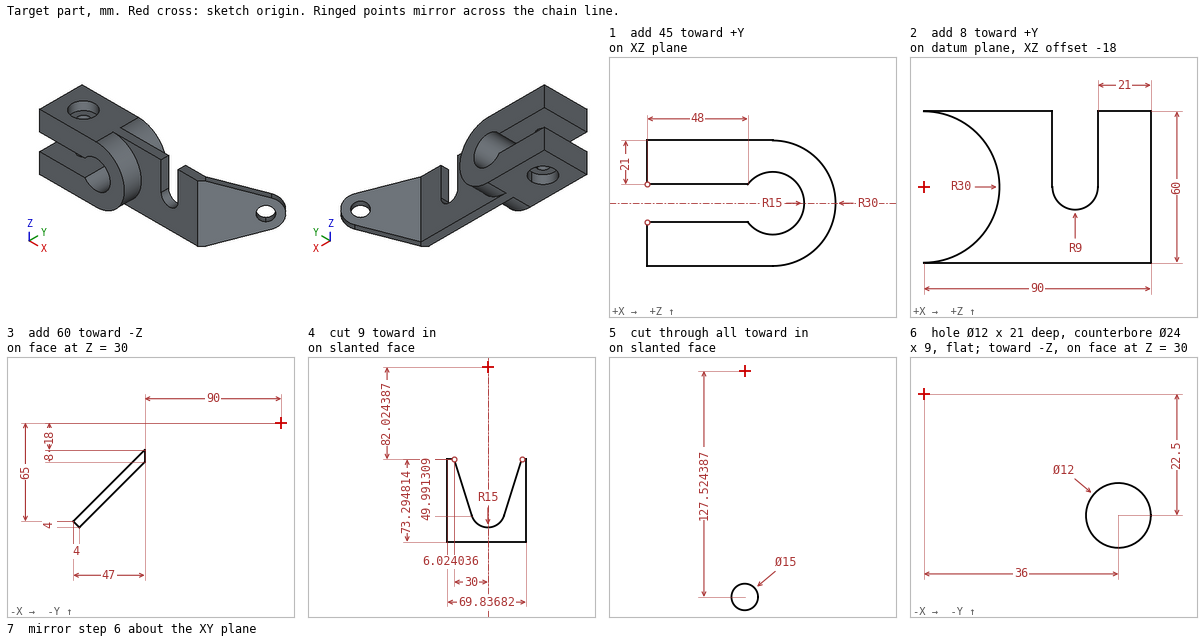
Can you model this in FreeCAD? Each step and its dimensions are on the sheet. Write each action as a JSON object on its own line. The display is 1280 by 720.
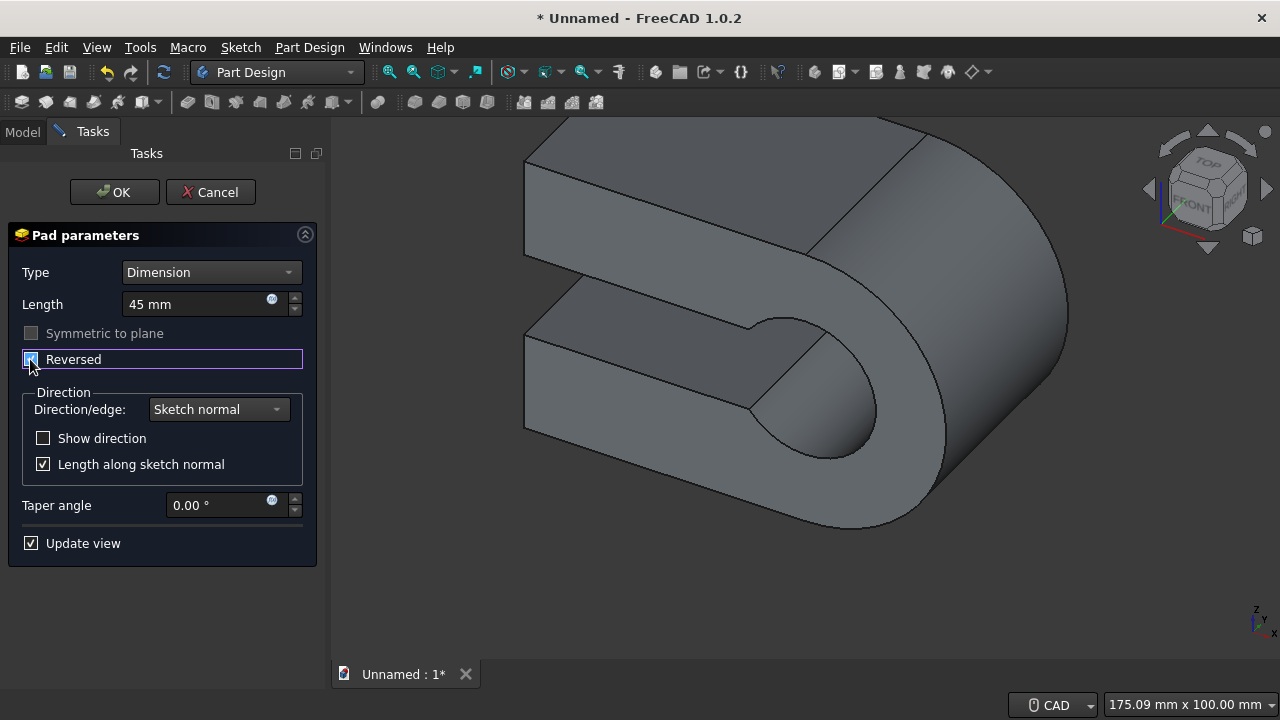
{"action": "left_click", "coordinate": [115, 192]}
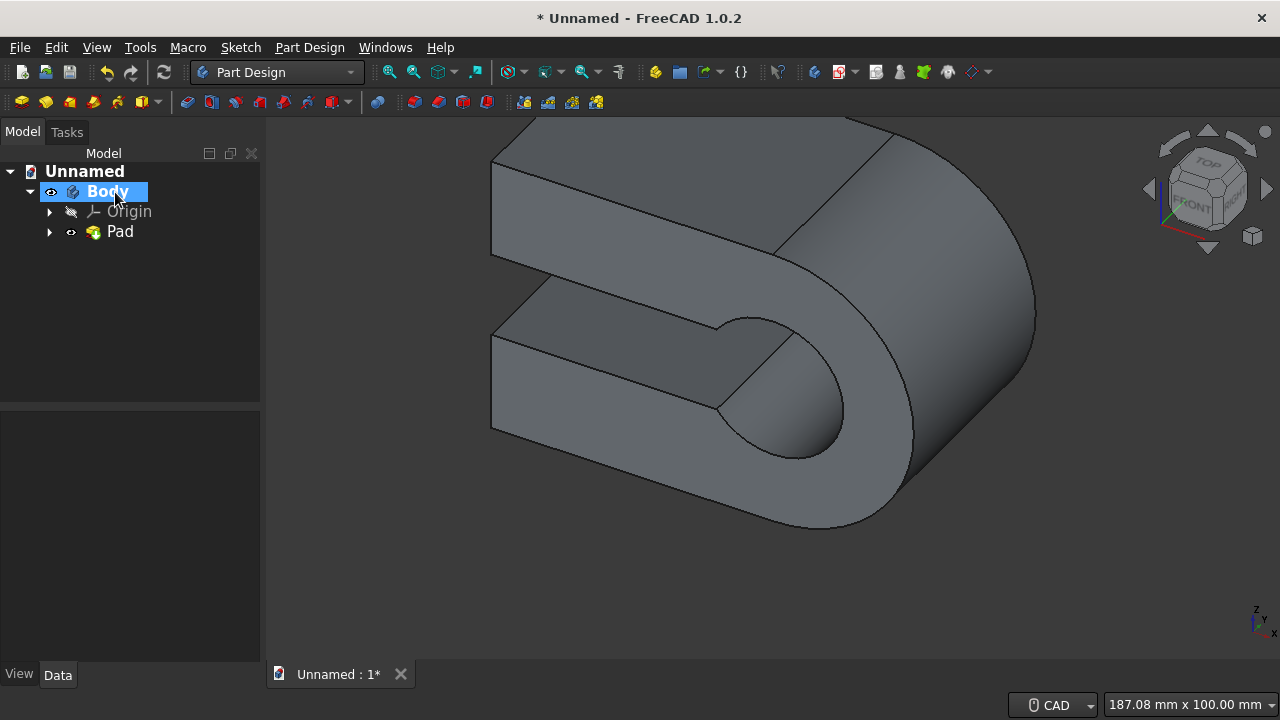
{"action": "left_click", "coordinate": [390, 72]}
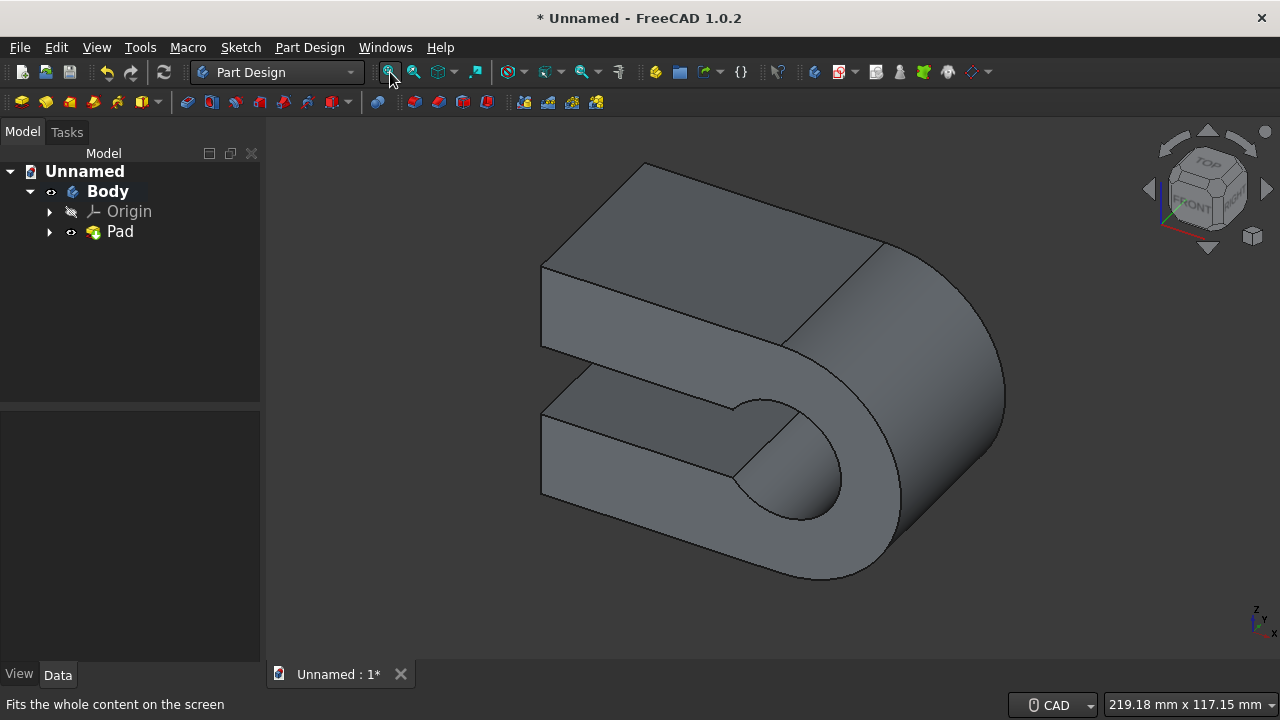
{"action": "left_click", "coordinate": [50, 212]}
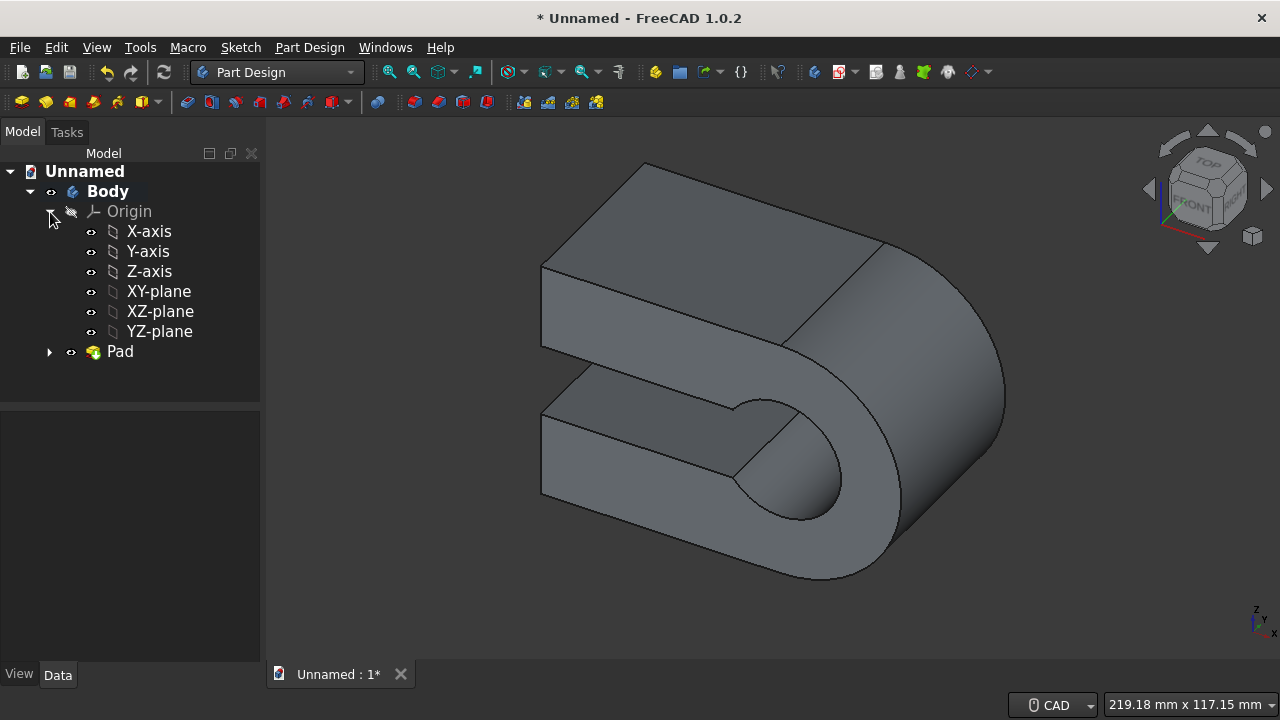
{"action": "left_click", "coordinate": [136, 312]}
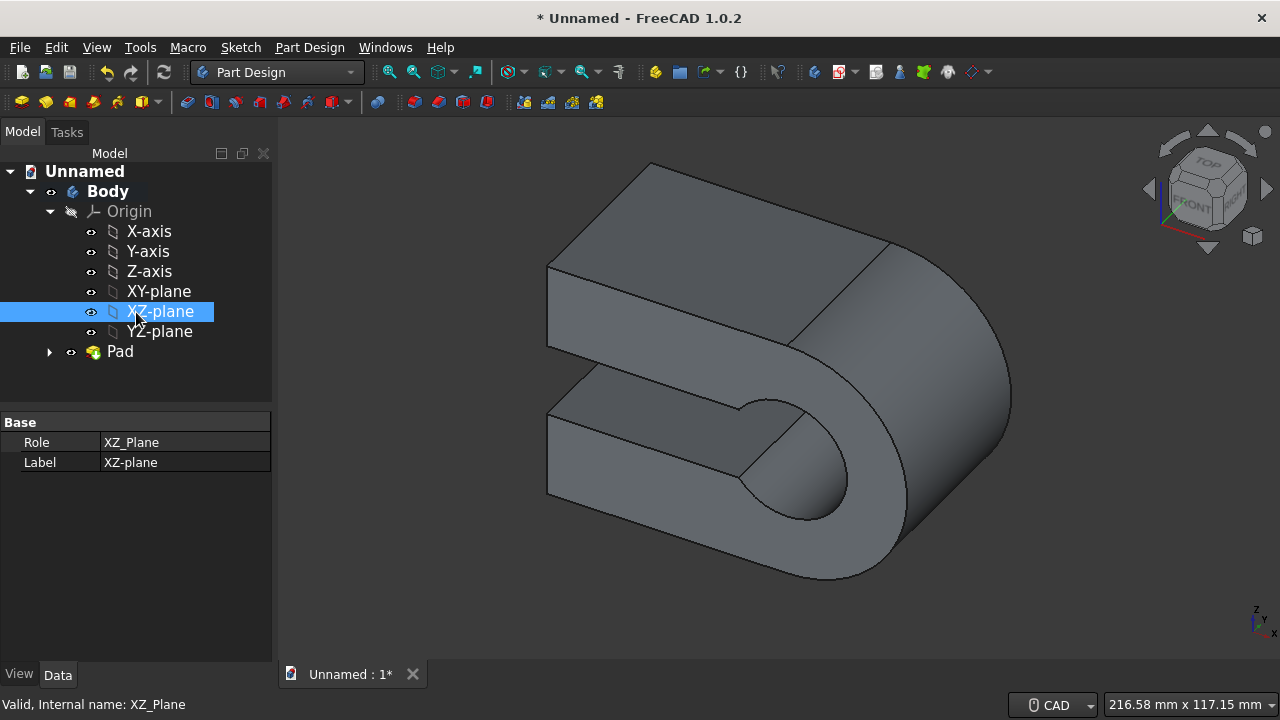
{"action": "left_click", "coordinate": [972, 72]}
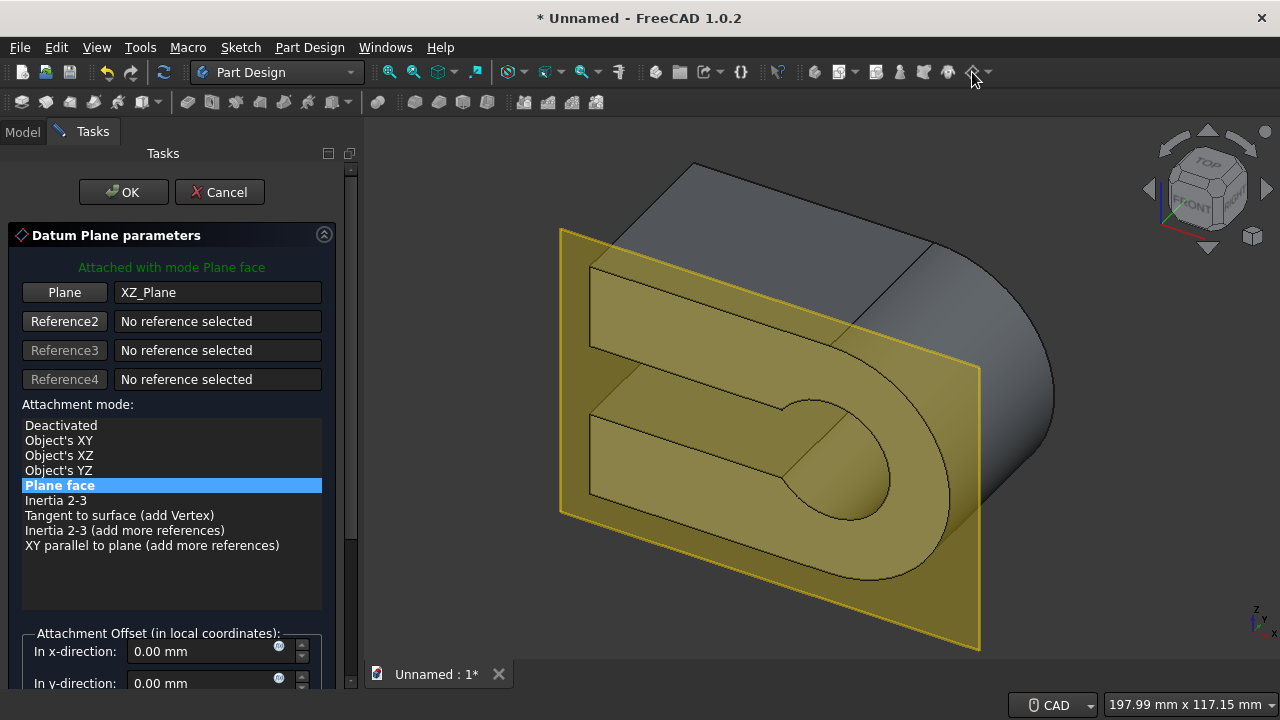
{"action": "scroll", "coordinate": [351, 426], "scroll_direction": "down", "scroll_amount": 2}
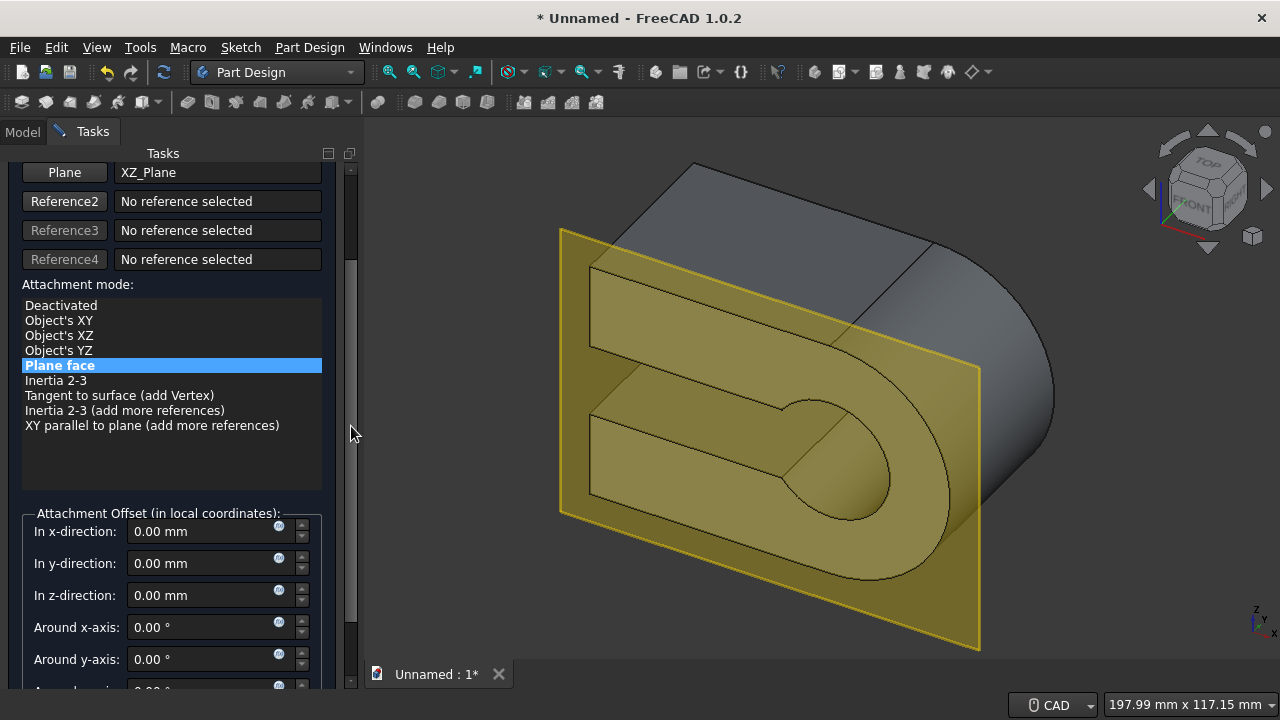
{"action": "triple_click", "coordinate": [210, 595]}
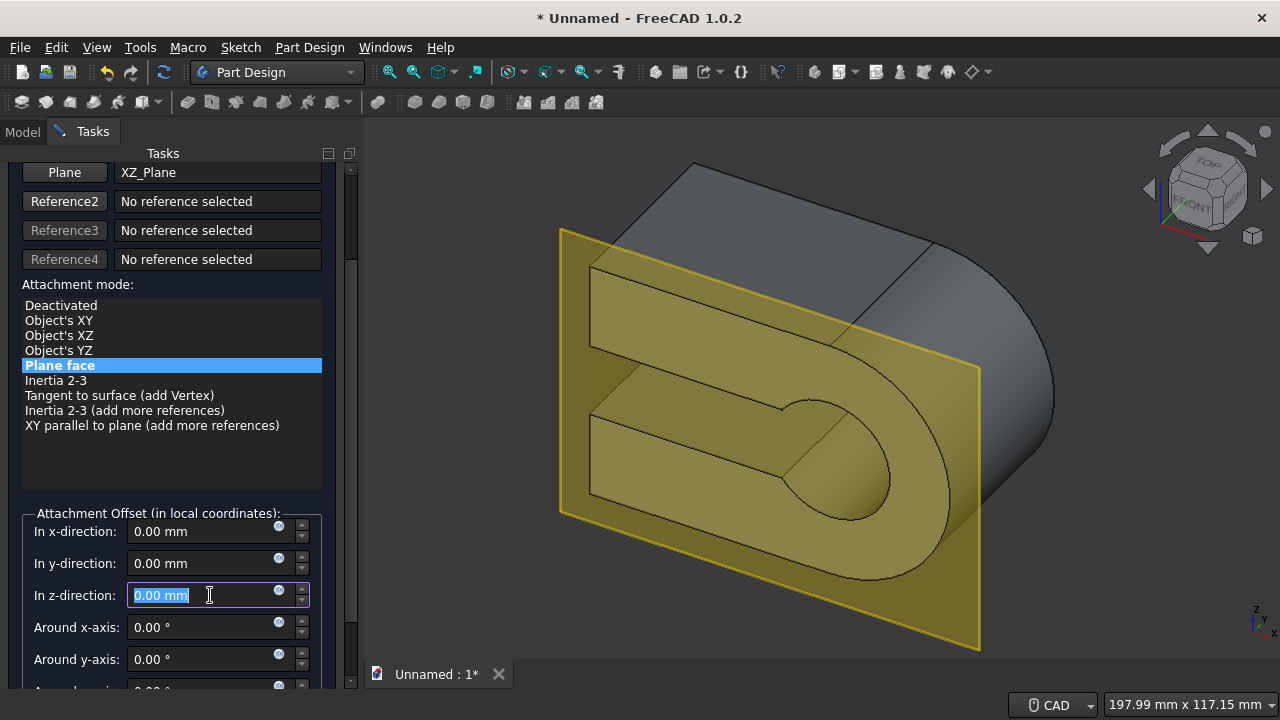
{"action": "type", "text": "-18"}
{"action": "key", "text": "Tab"}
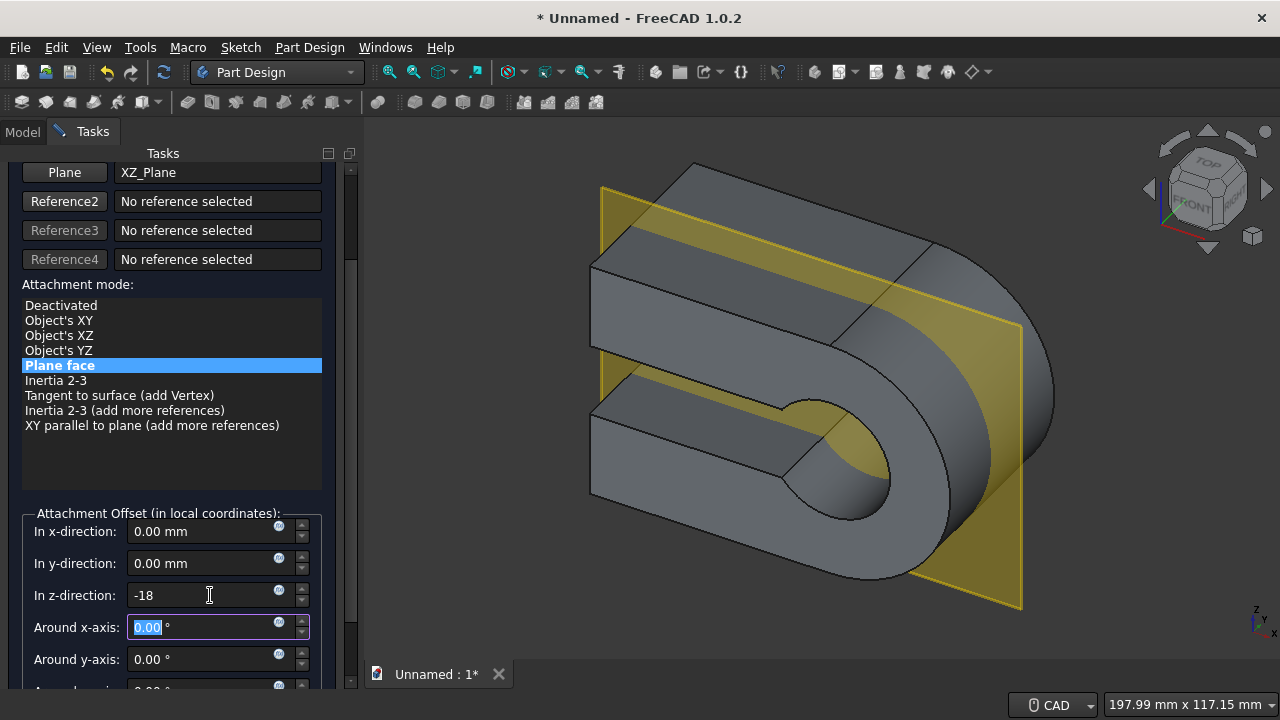
{"action": "scroll", "coordinate": [351, 426], "scroll_direction": "up", "scroll_amount": 3}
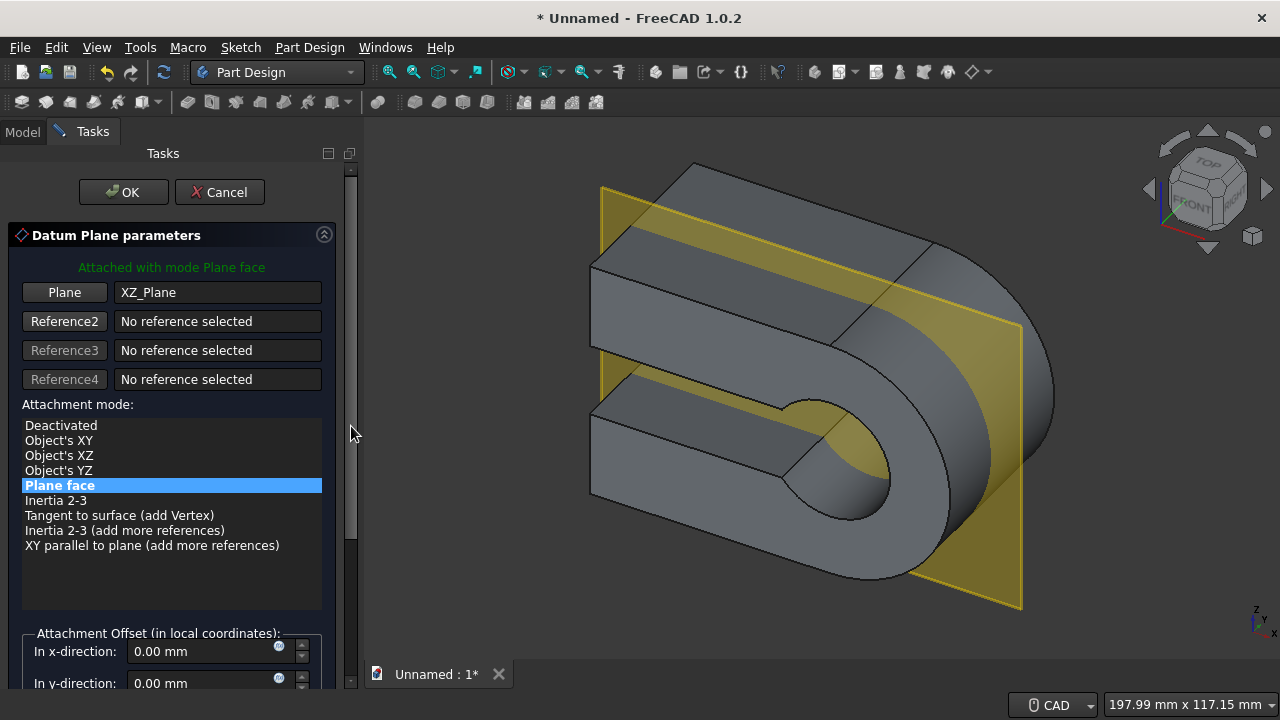
{"action": "left_click", "coordinate": [124, 192]}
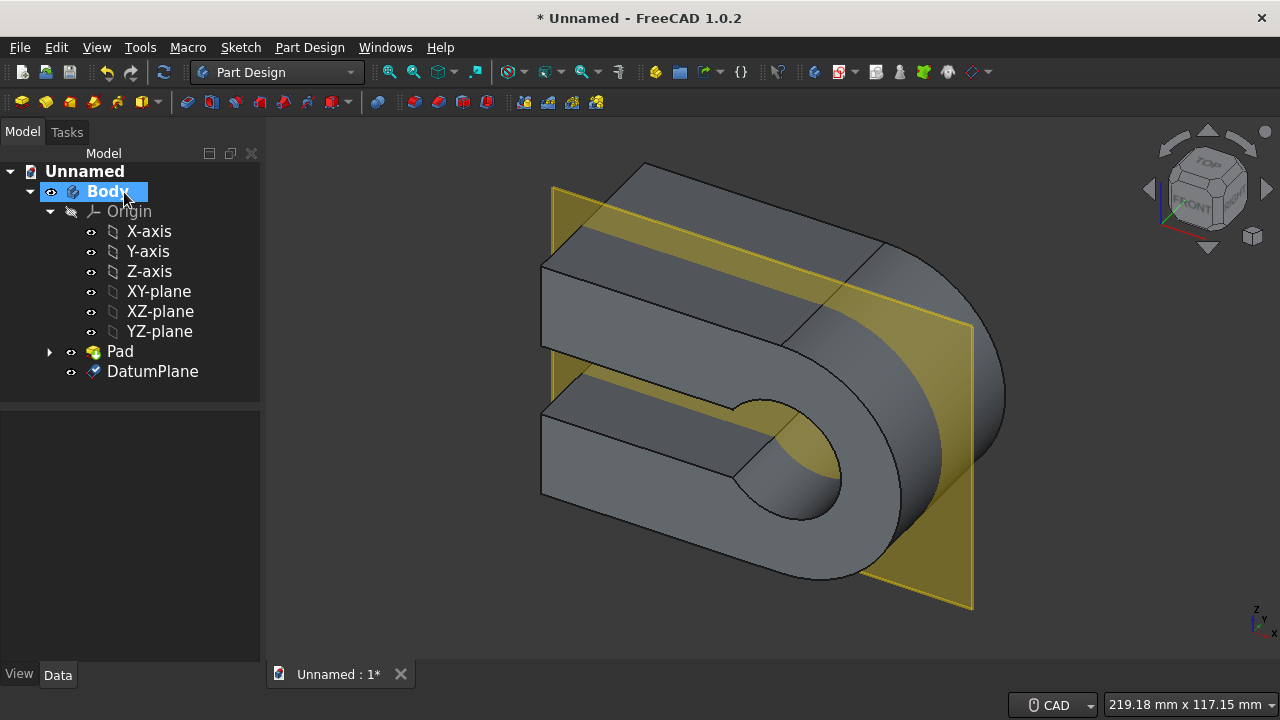
{"action": "left_click", "coordinate": [116, 372]}